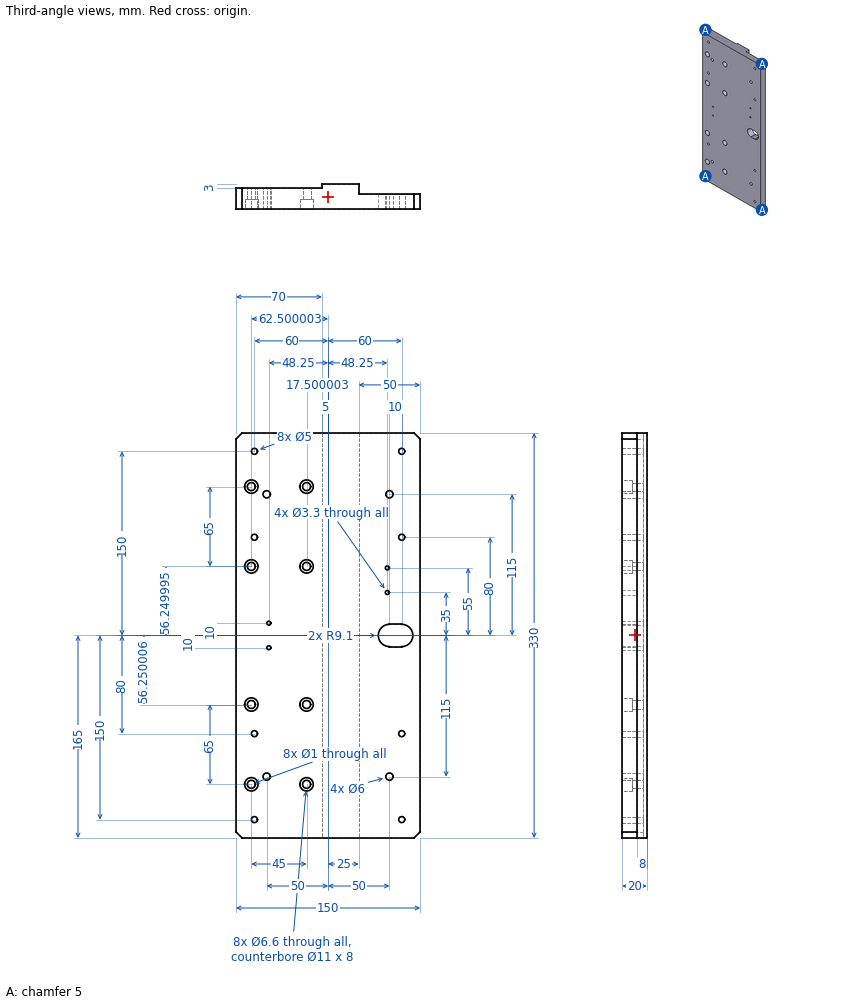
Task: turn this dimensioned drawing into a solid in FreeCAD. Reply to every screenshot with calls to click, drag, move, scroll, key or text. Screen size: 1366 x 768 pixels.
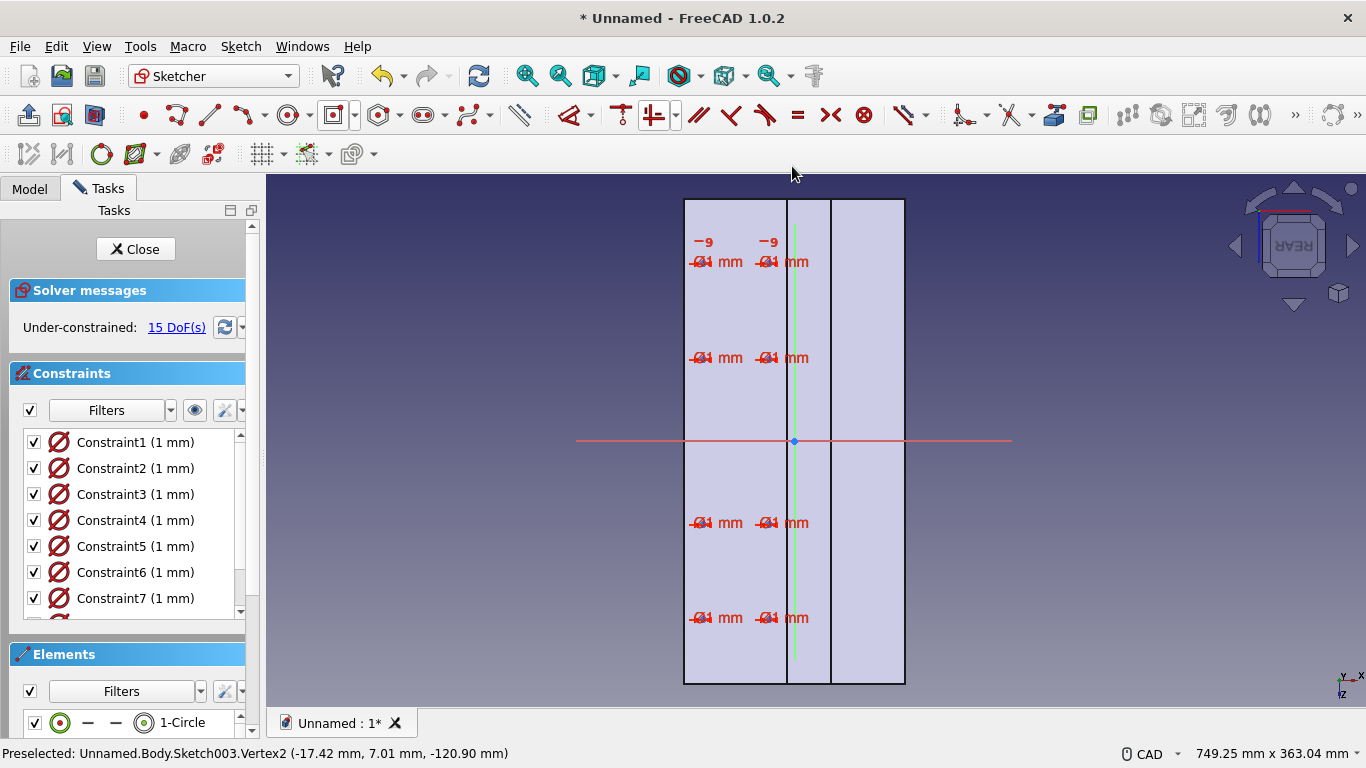
click(703, 264)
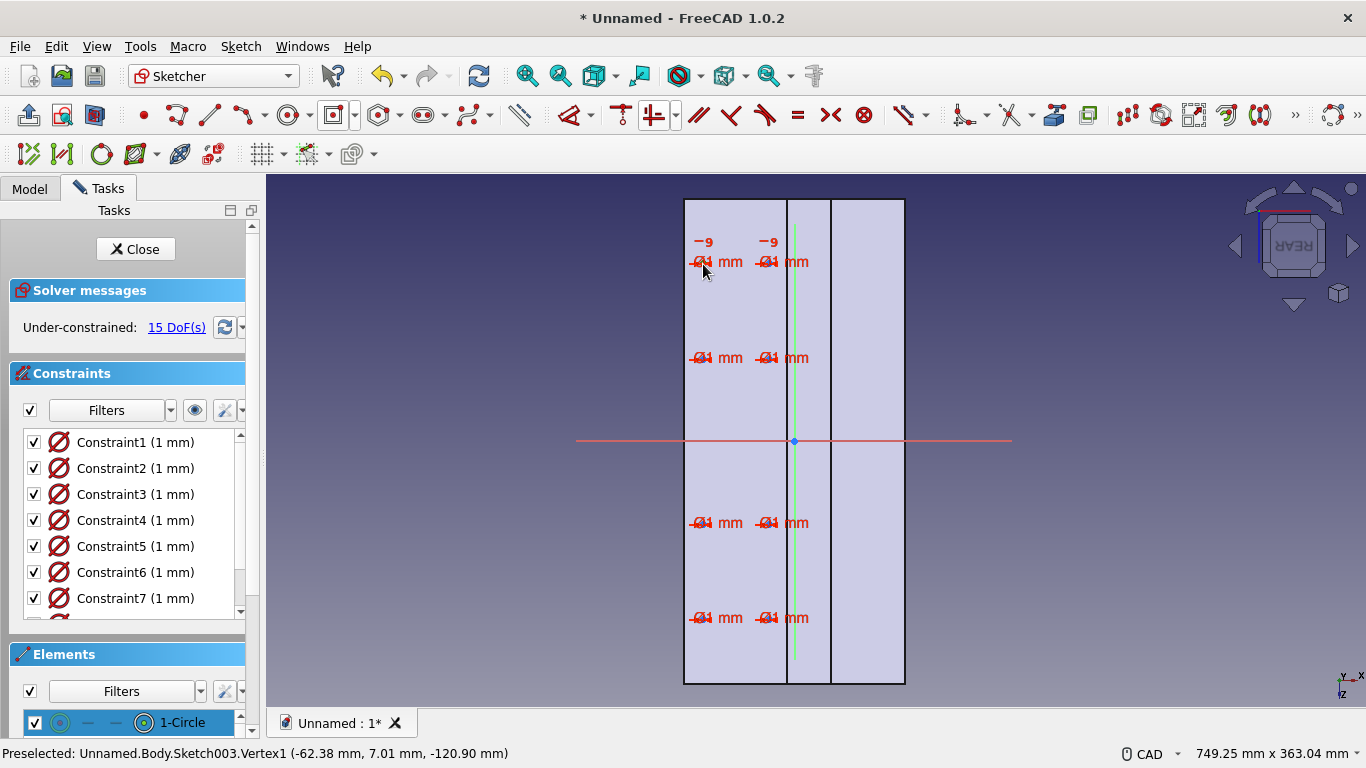
click(703, 360)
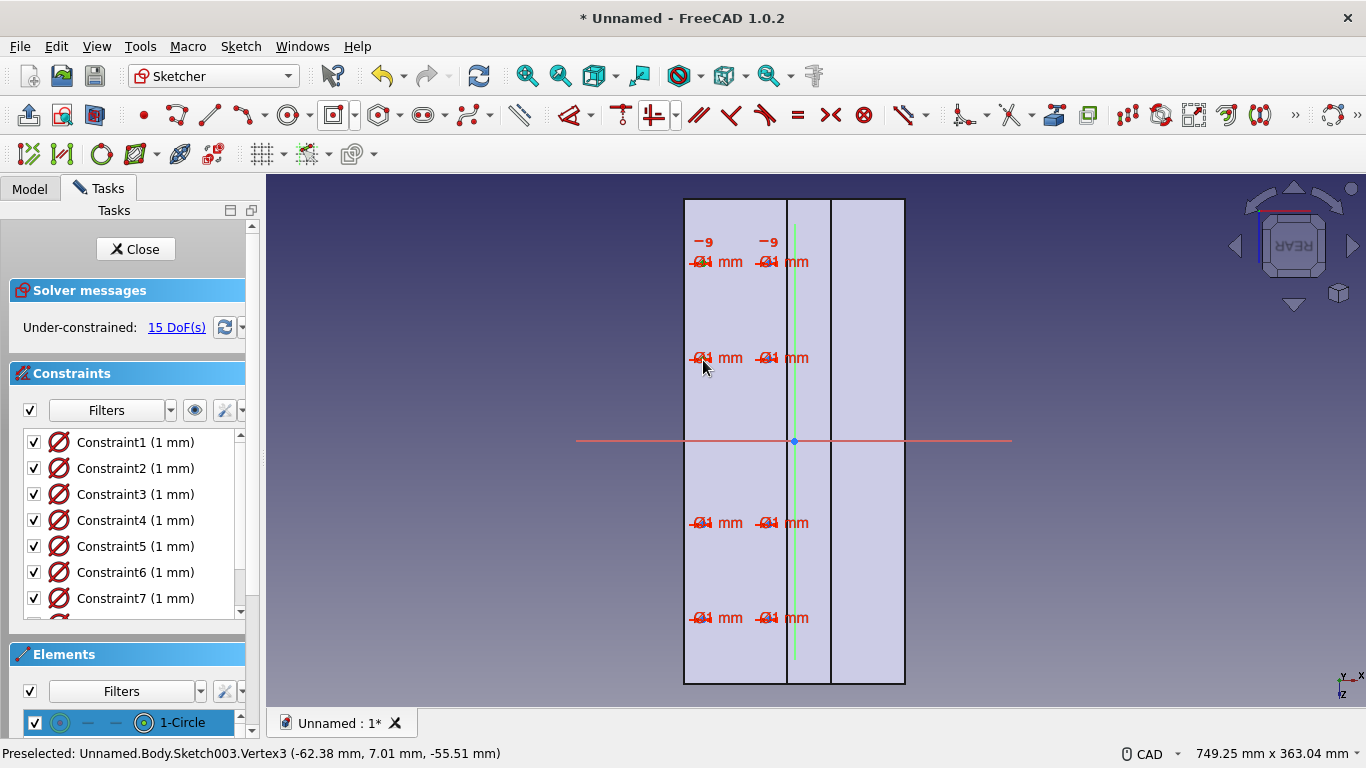
click(676, 116)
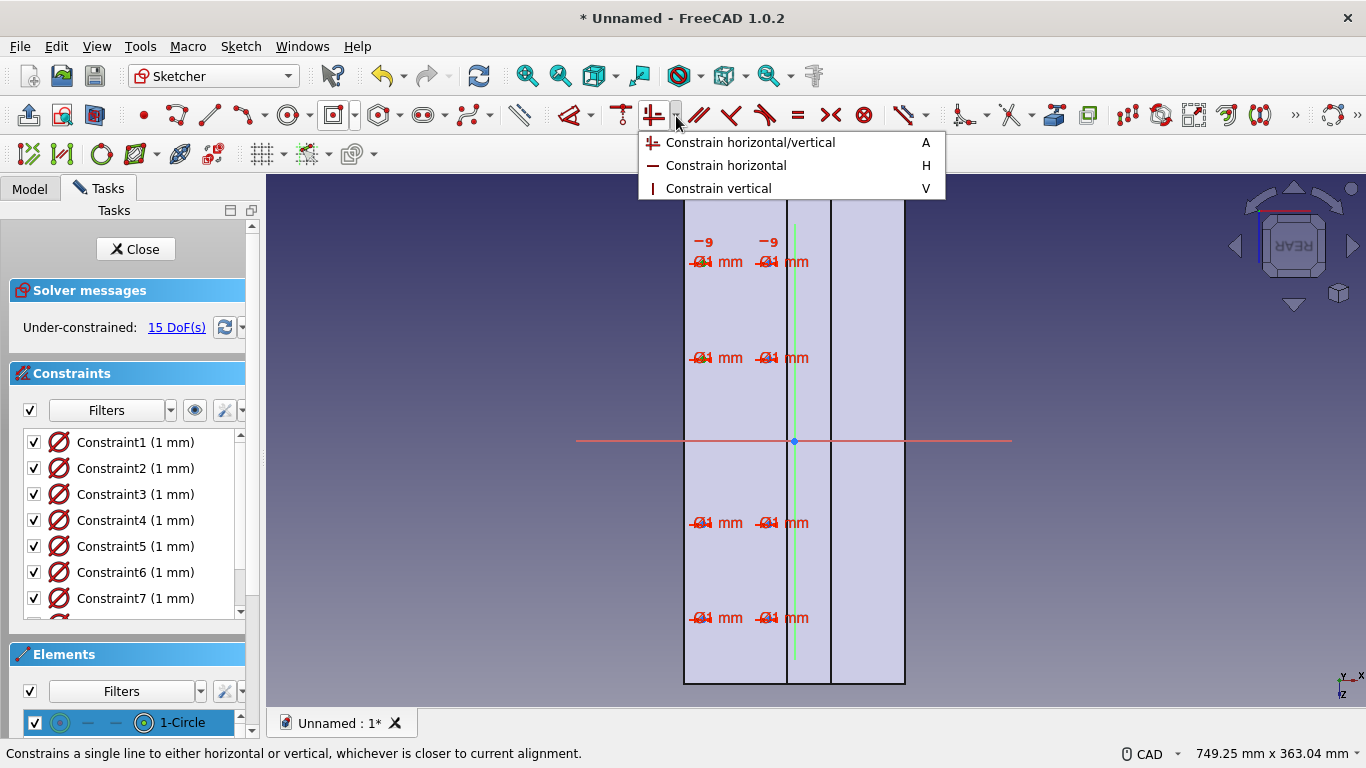
click(792, 188)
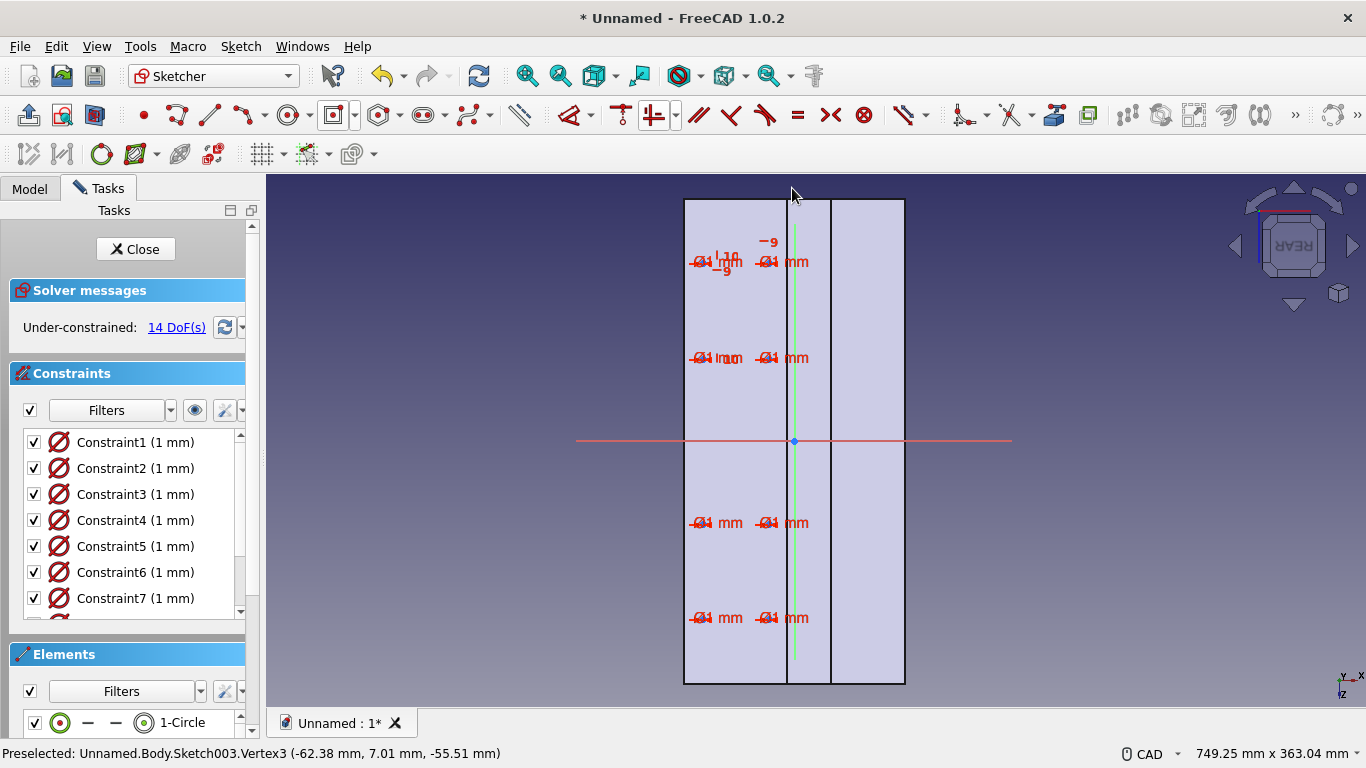
click(769, 264)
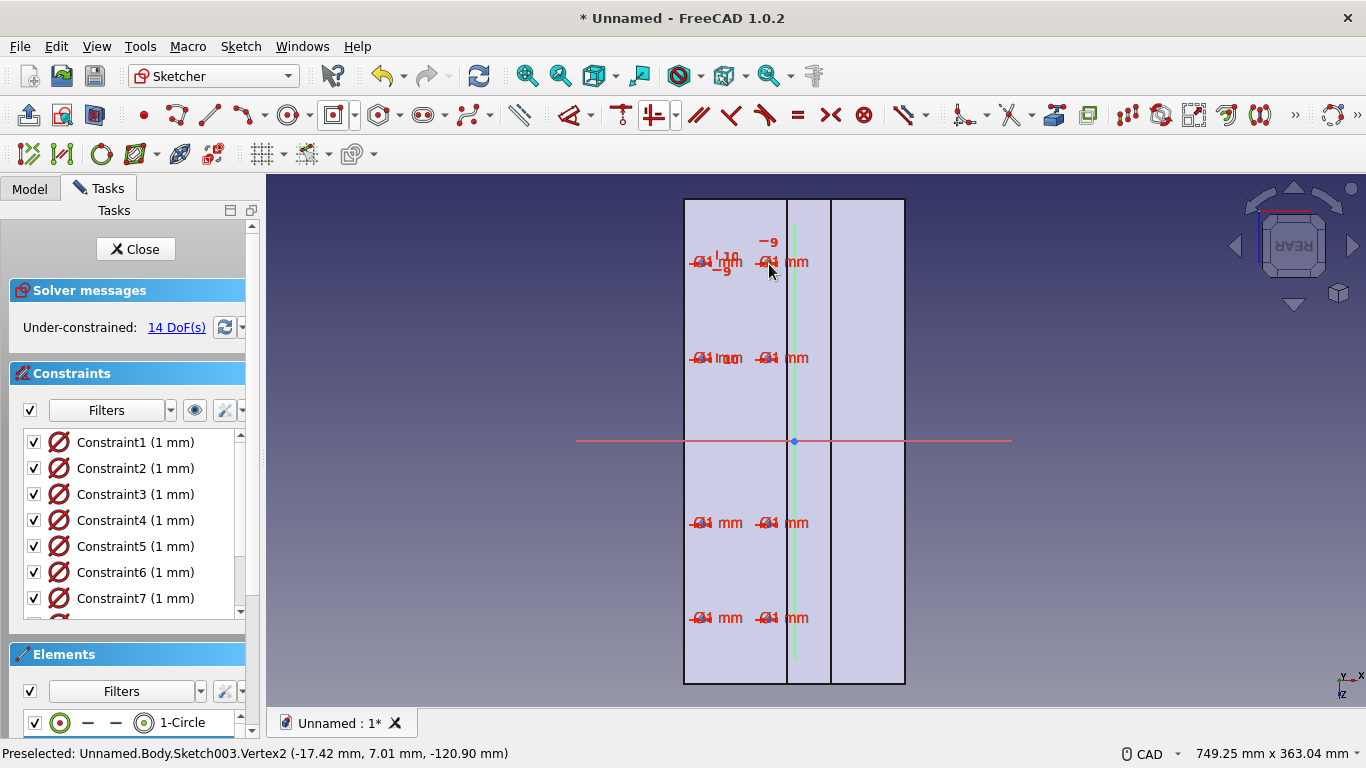
click(769, 360)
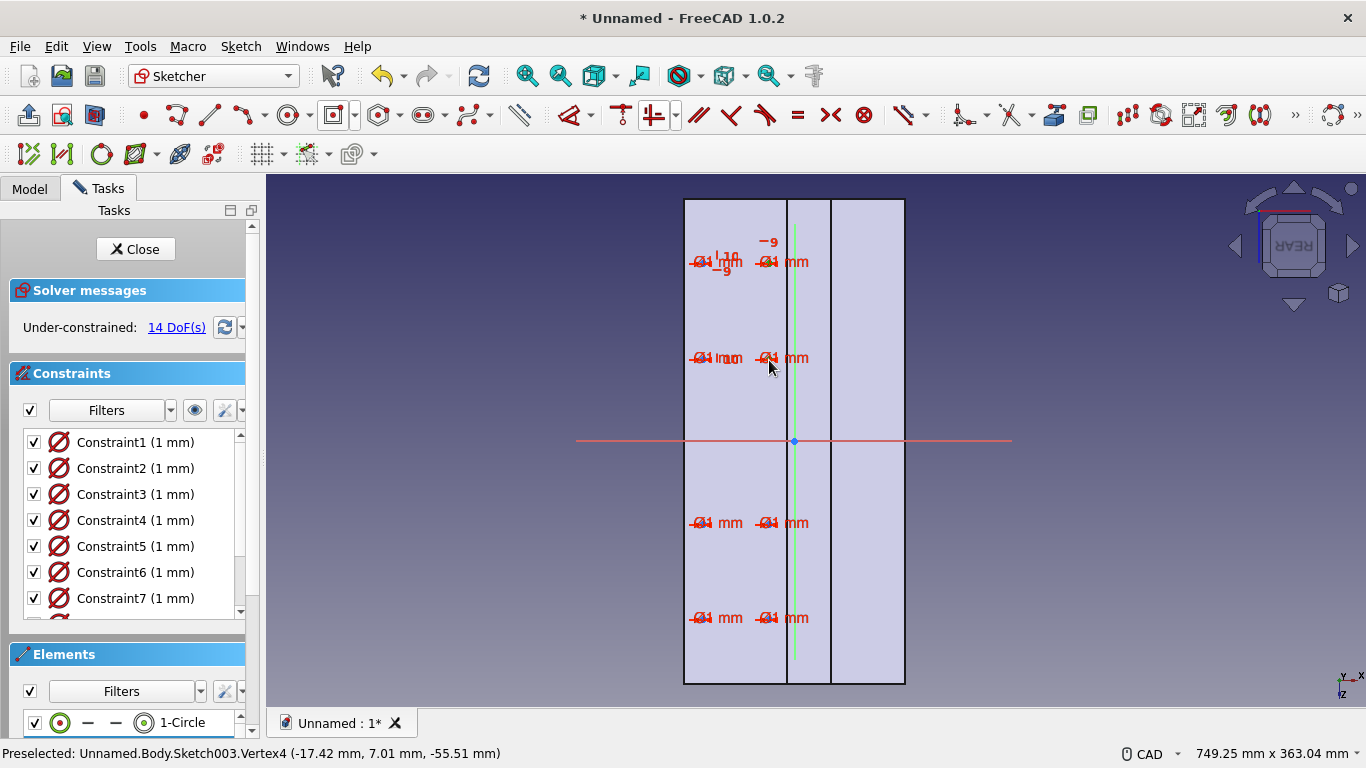
click(676, 116)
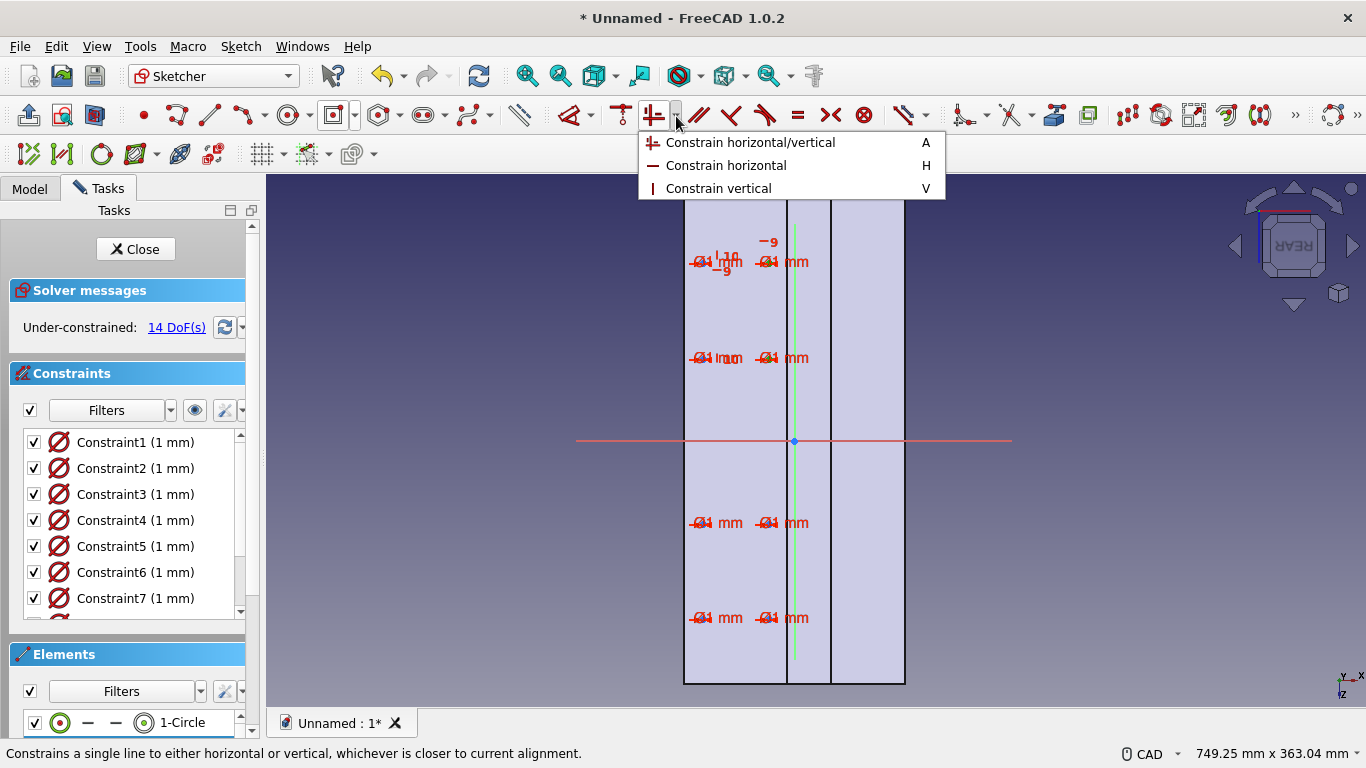
click(792, 188)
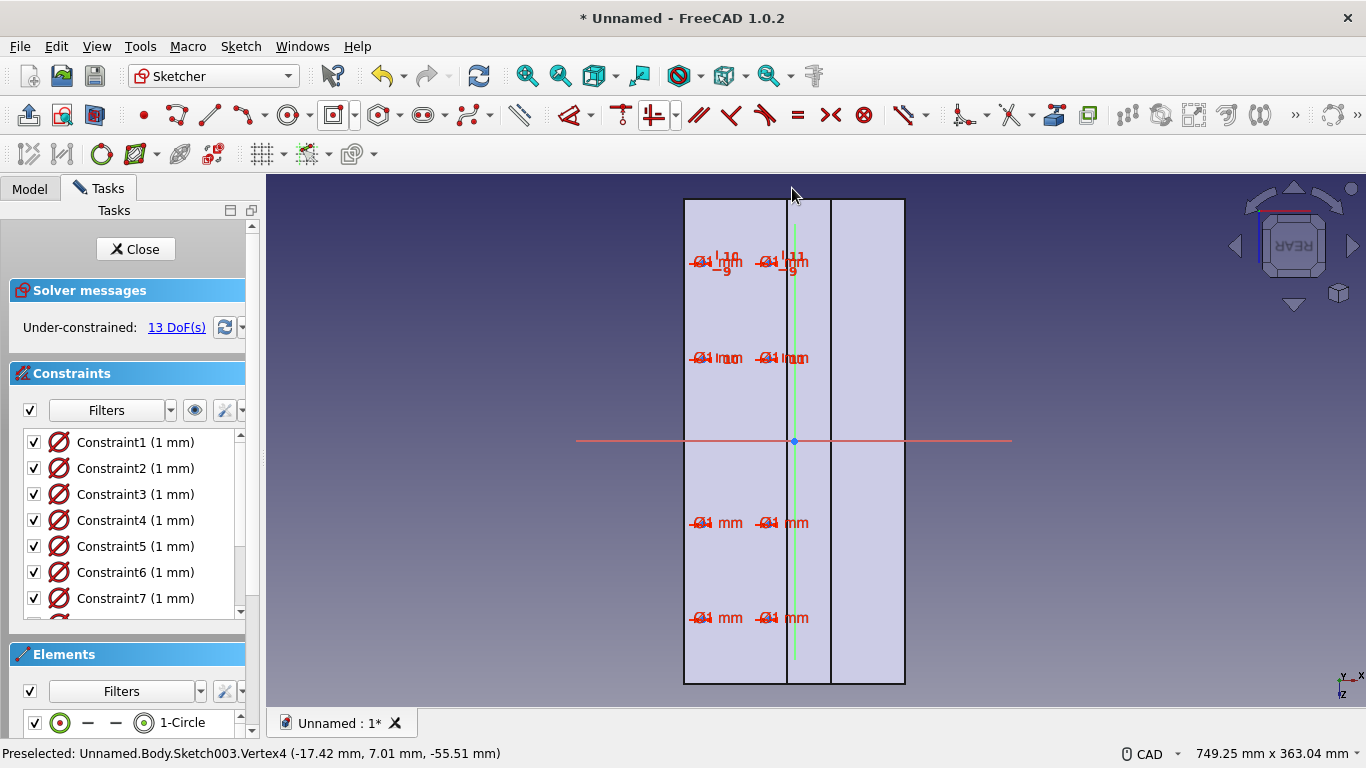
click(703, 360)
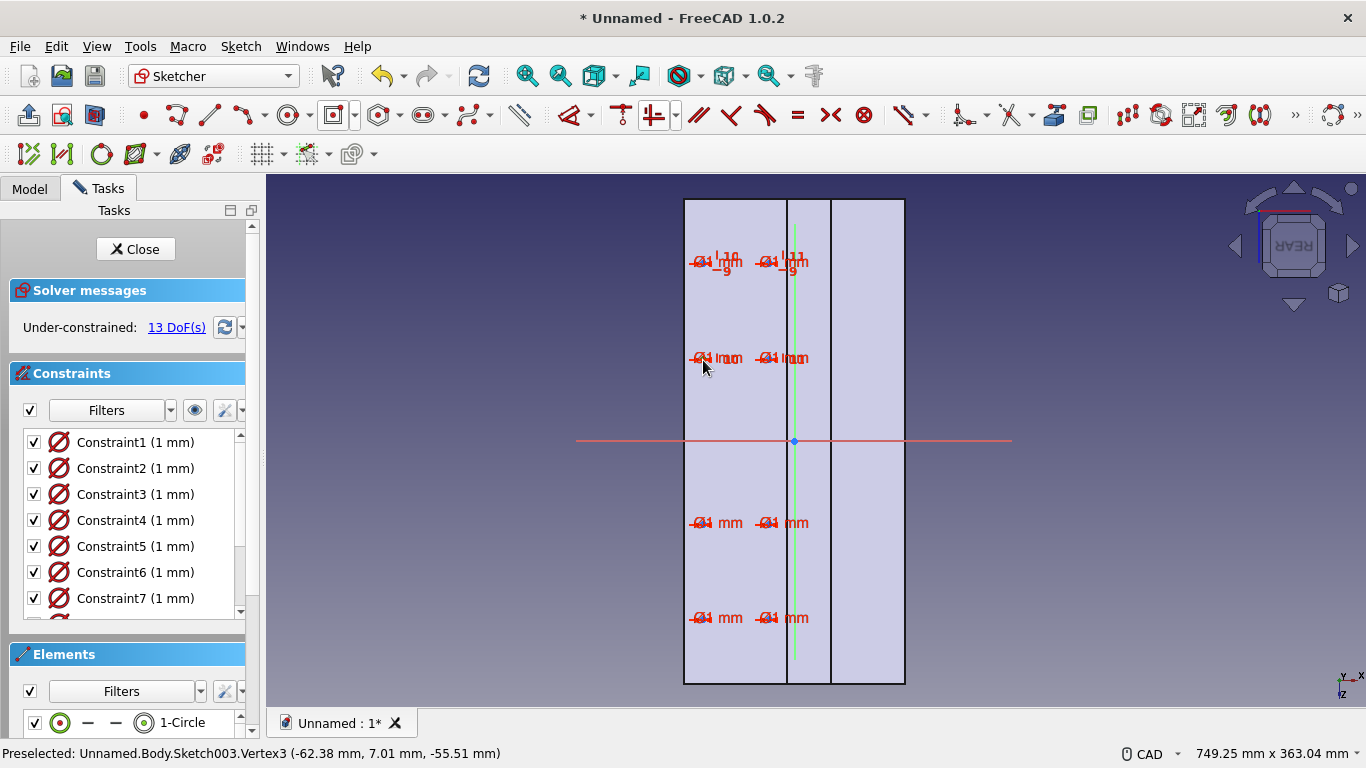
click(769, 360)